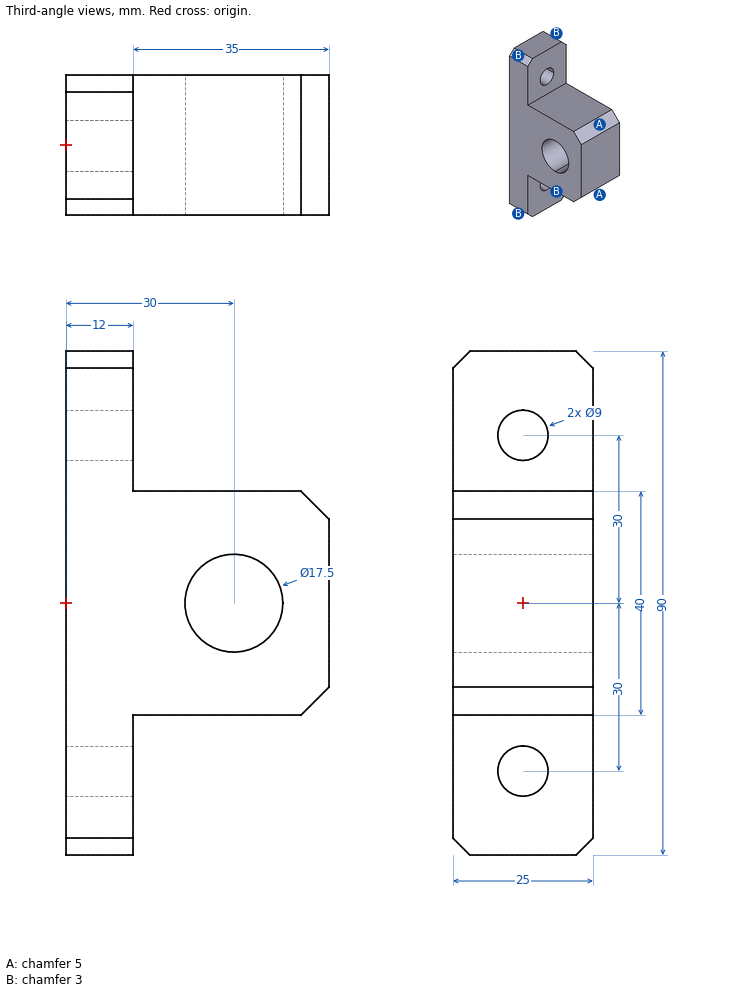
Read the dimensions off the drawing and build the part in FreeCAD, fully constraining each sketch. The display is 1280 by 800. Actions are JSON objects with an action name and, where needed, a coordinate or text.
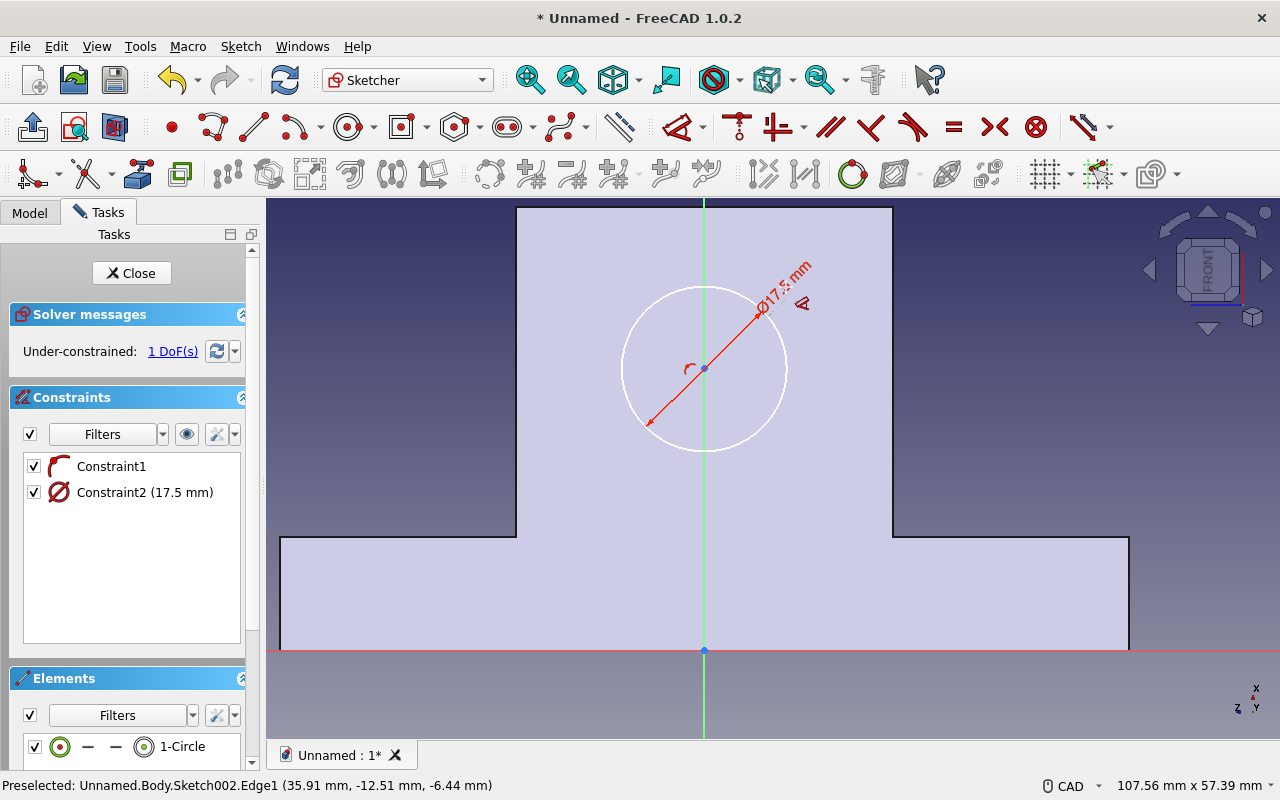
{"action": "left_click", "coordinate": [704, 369]}
{"action": "left_click", "coordinate": [738, 510]}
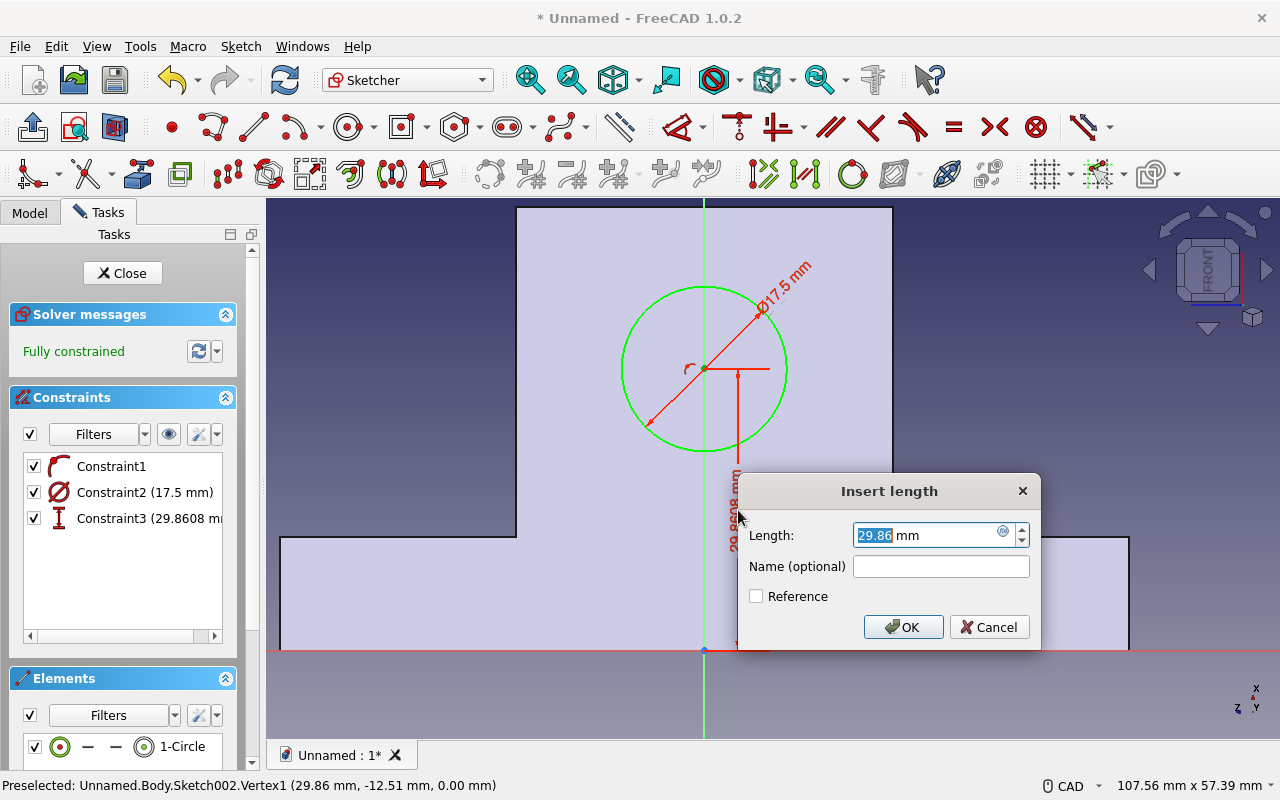
{"action": "type", "text": "30"}
{"action": "key", "text": "Return"}
{"action": "key", "text": "Escape"}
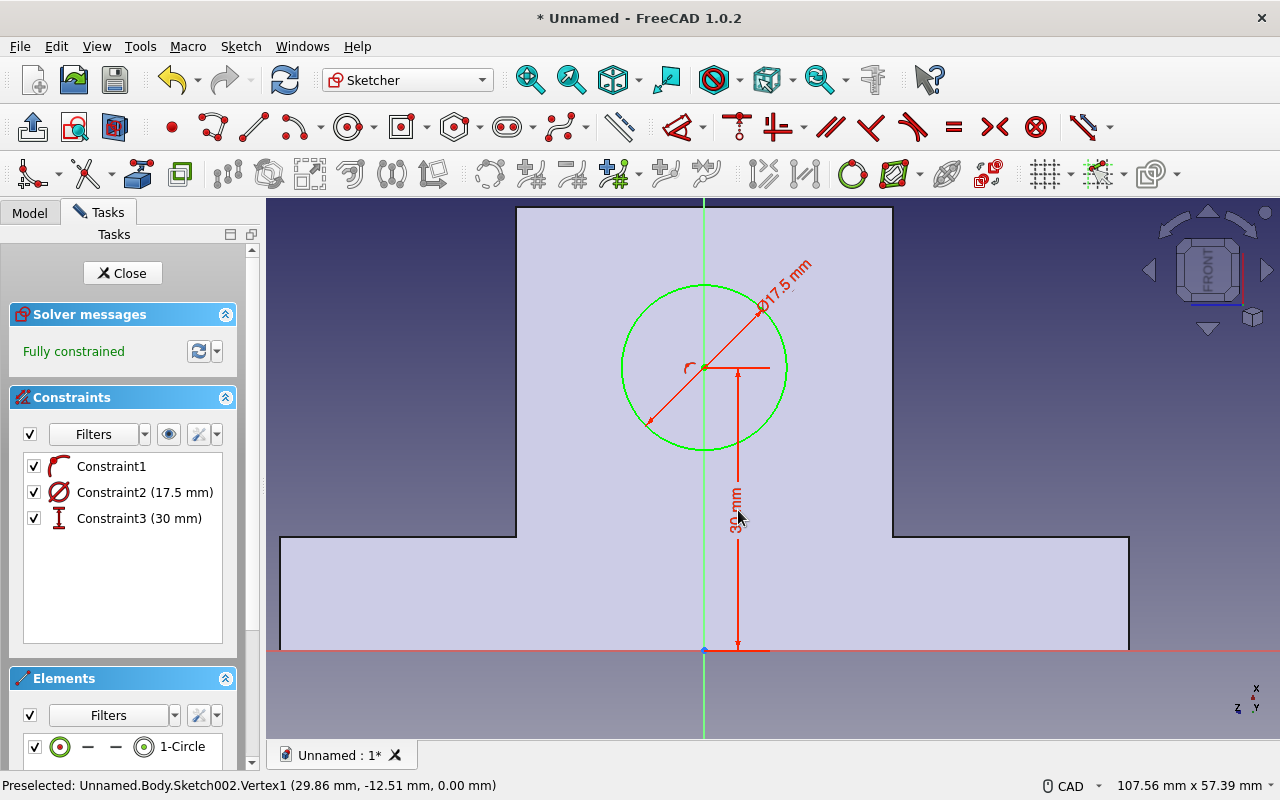
{"action": "left_click", "coordinate": [123, 273]}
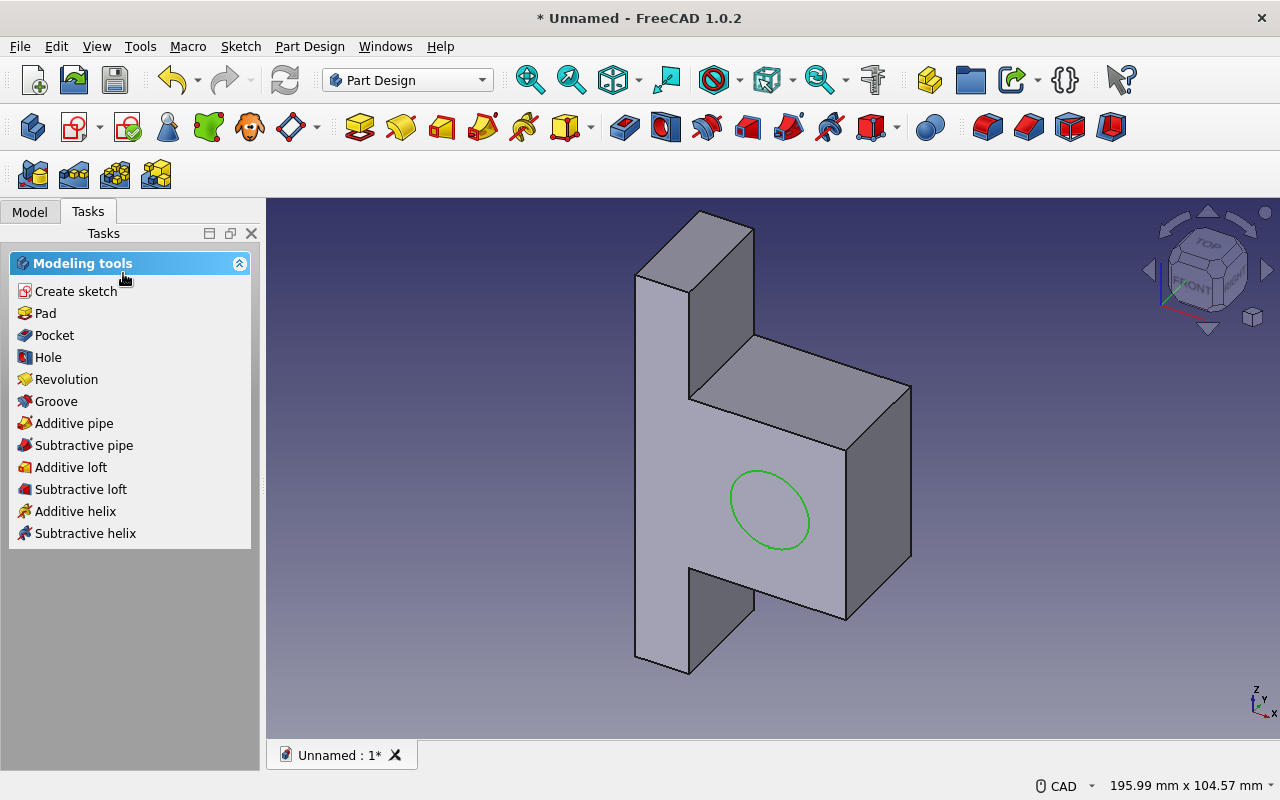
{"action": "left_click", "coordinate": [625, 128]}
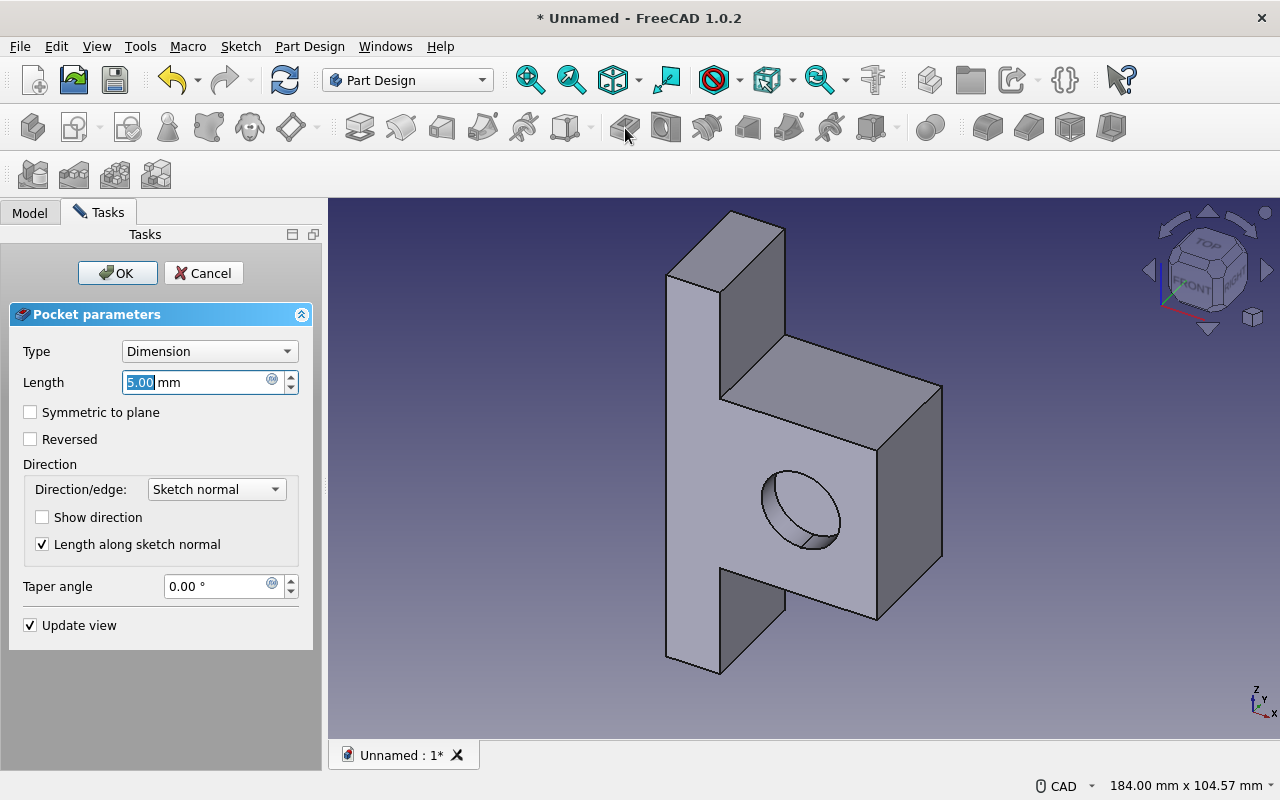
{"action": "left_click", "coordinate": [210, 352]}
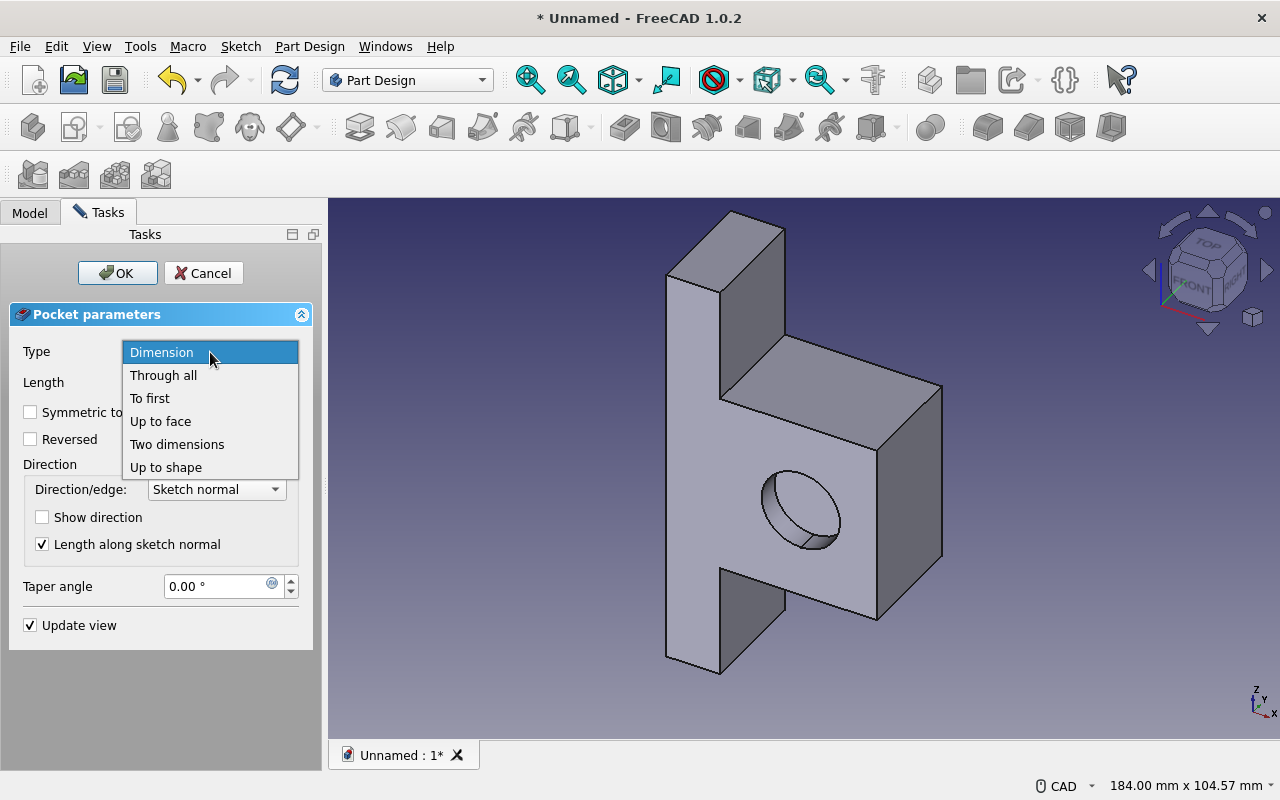
{"action": "left_click", "coordinate": [208, 376]}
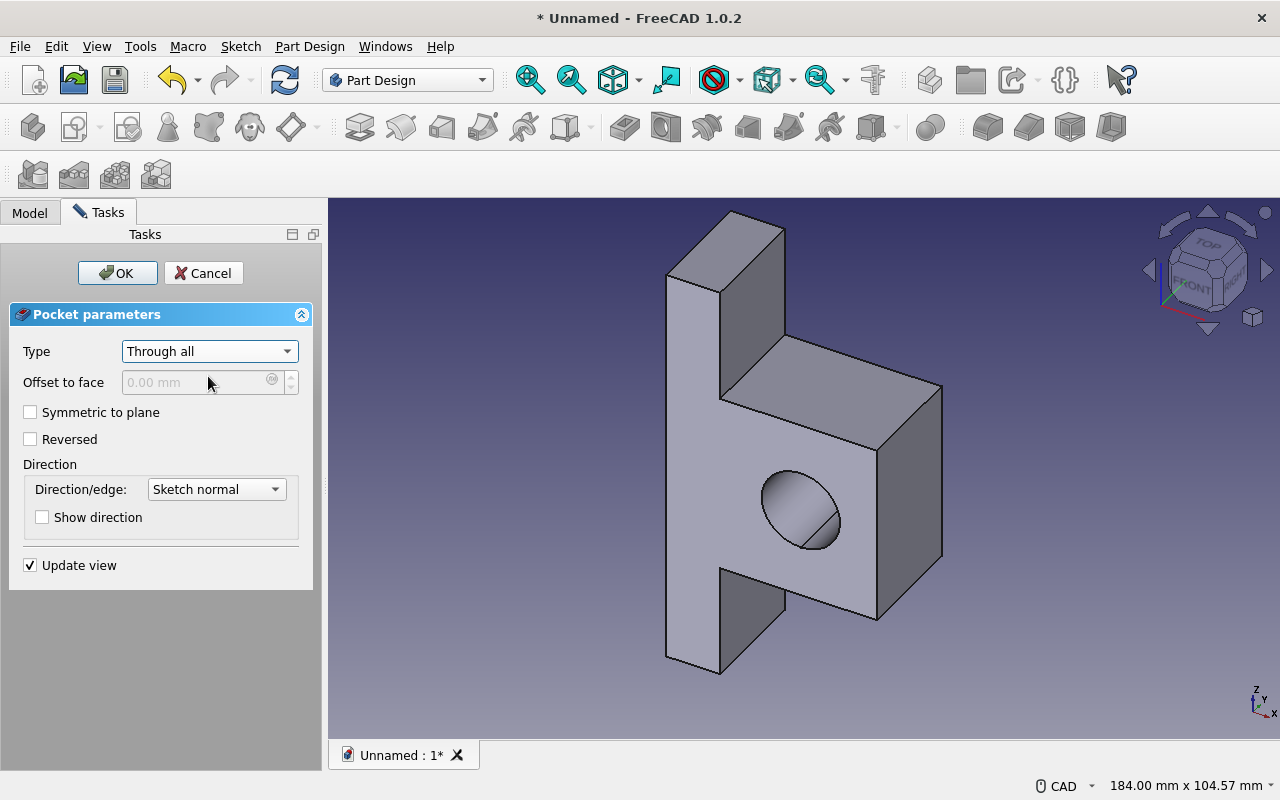
{"action": "left_click", "coordinate": [118, 273]}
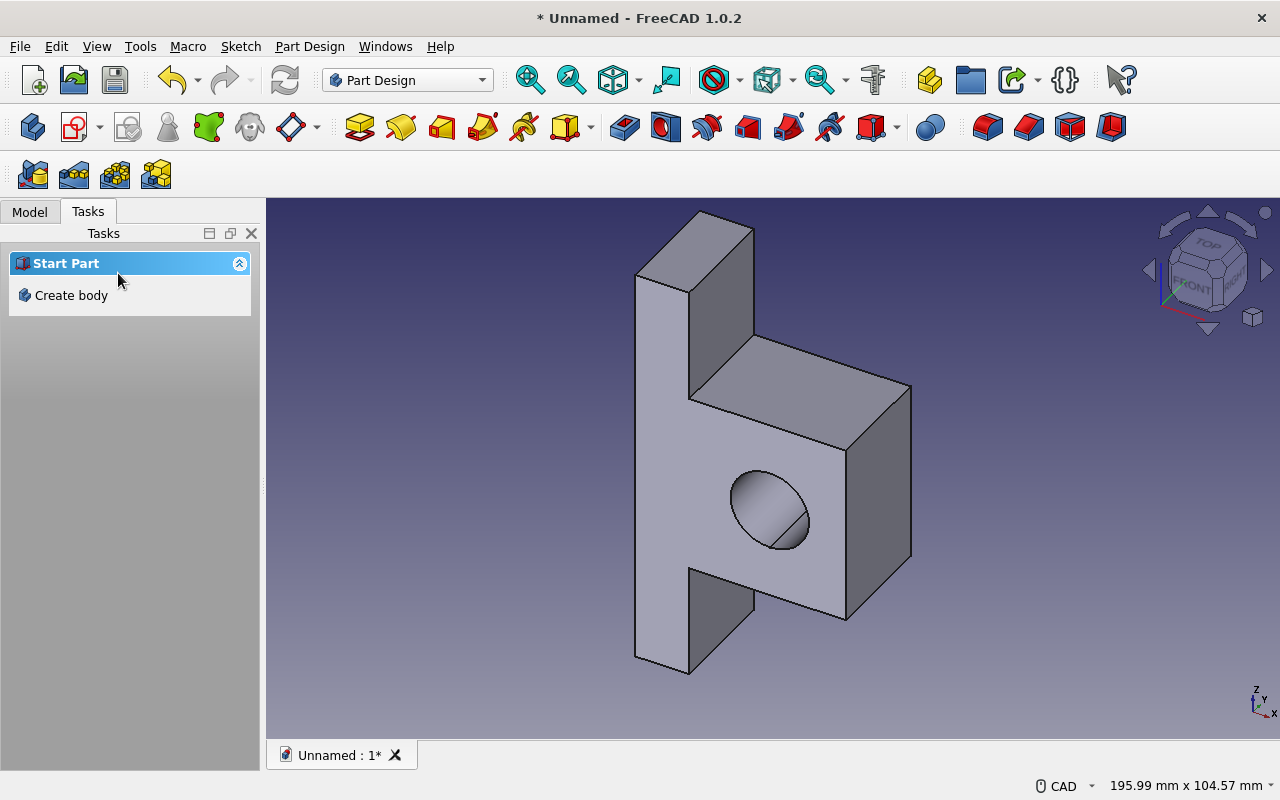
{"action": "left_click", "coordinate": [721, 313]}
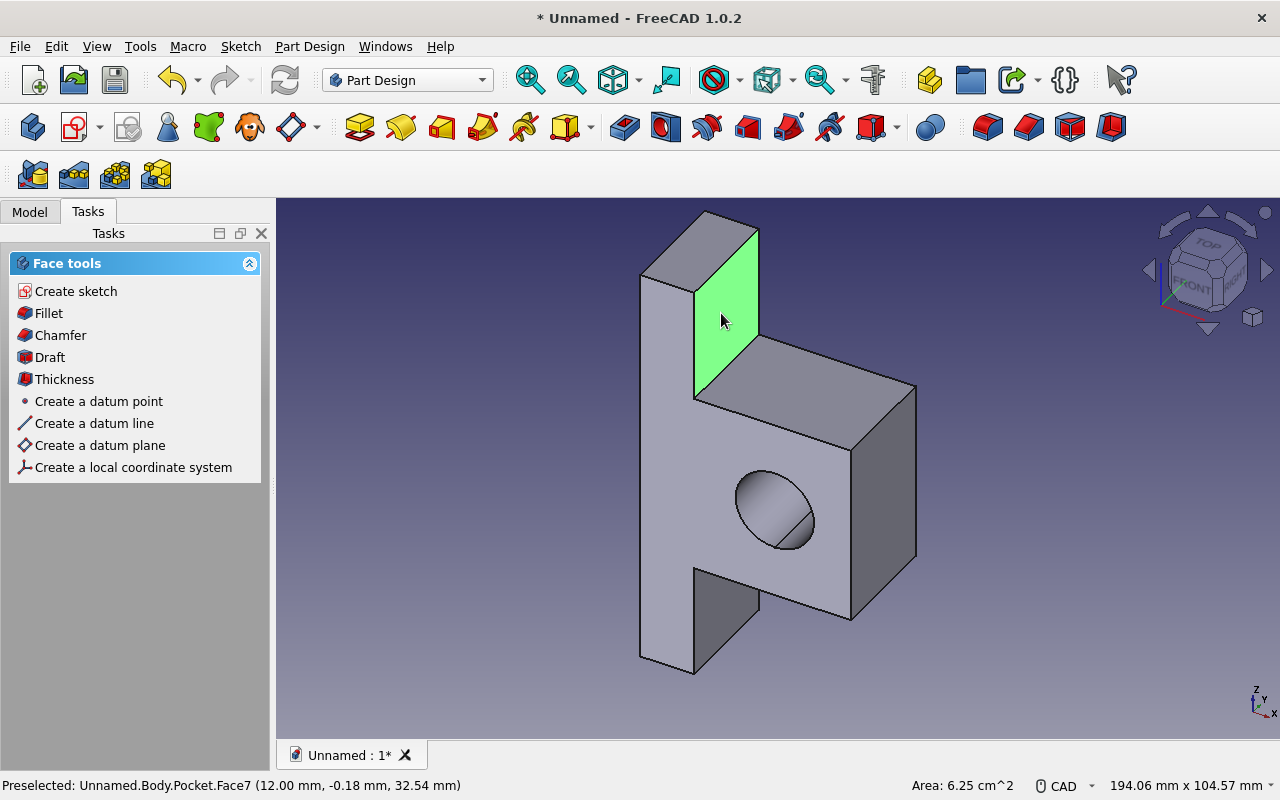
{"action": "left_click", "coordinate": [74, 128]}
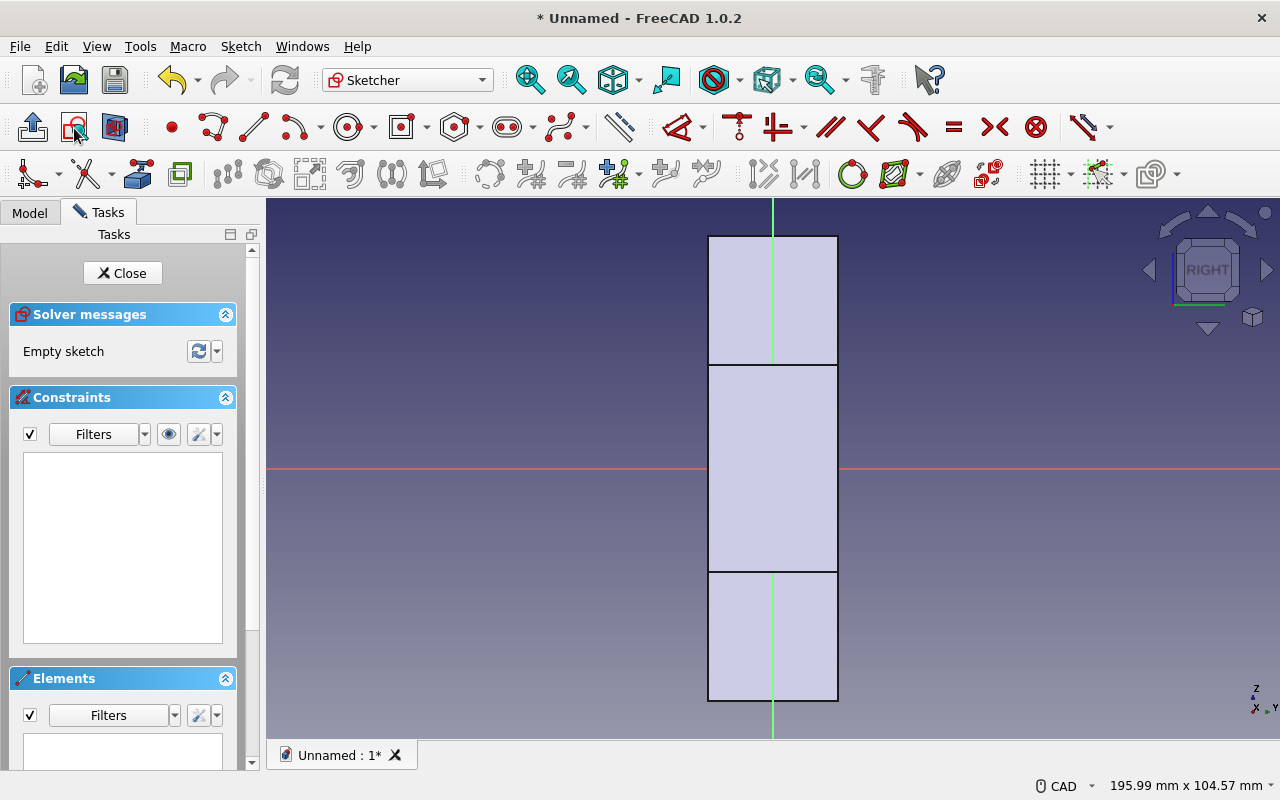
{"action": "left_click", "coordinate": [348, 128]}